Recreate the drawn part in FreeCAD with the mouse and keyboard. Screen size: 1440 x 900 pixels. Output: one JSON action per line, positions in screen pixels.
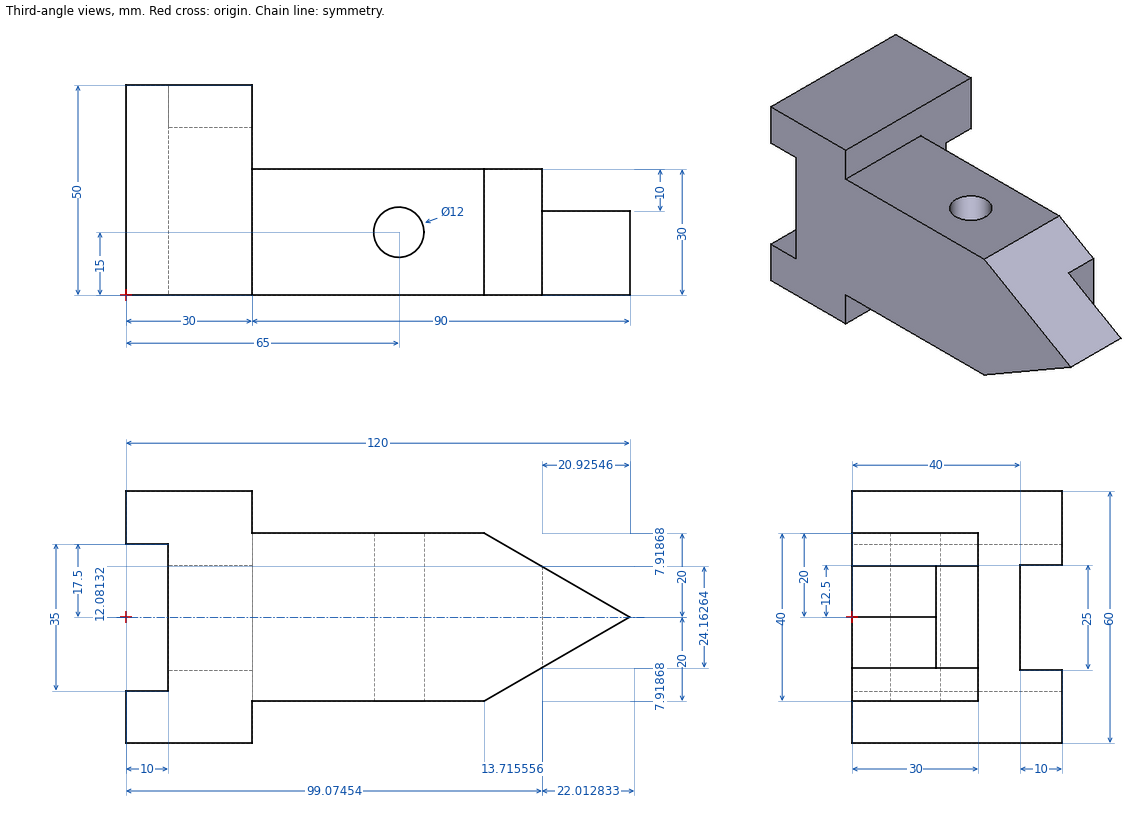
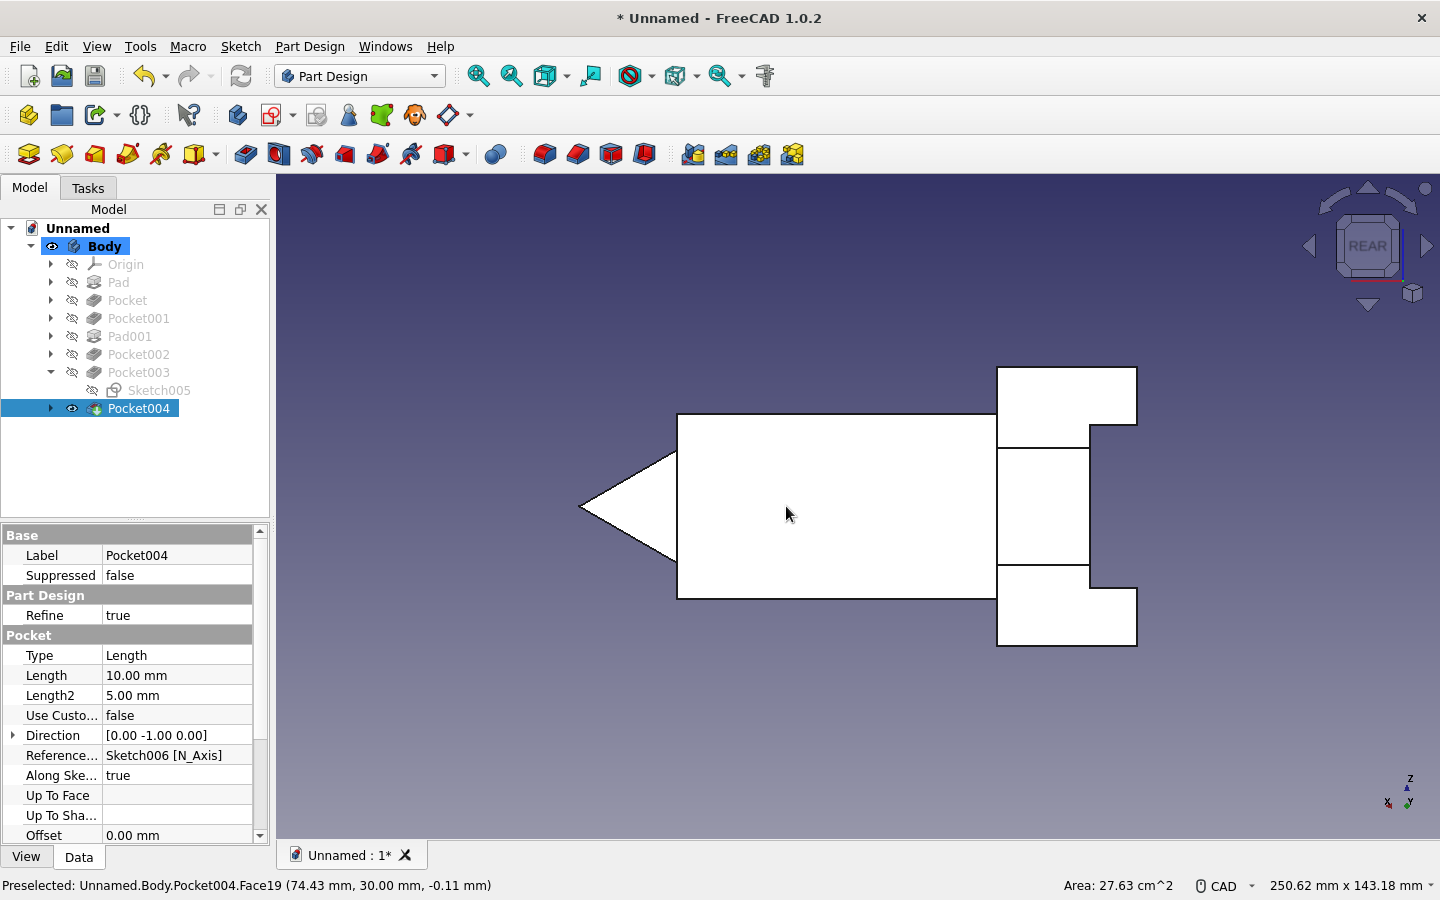
{"action": "left_click", "coordinate": [270, 116]}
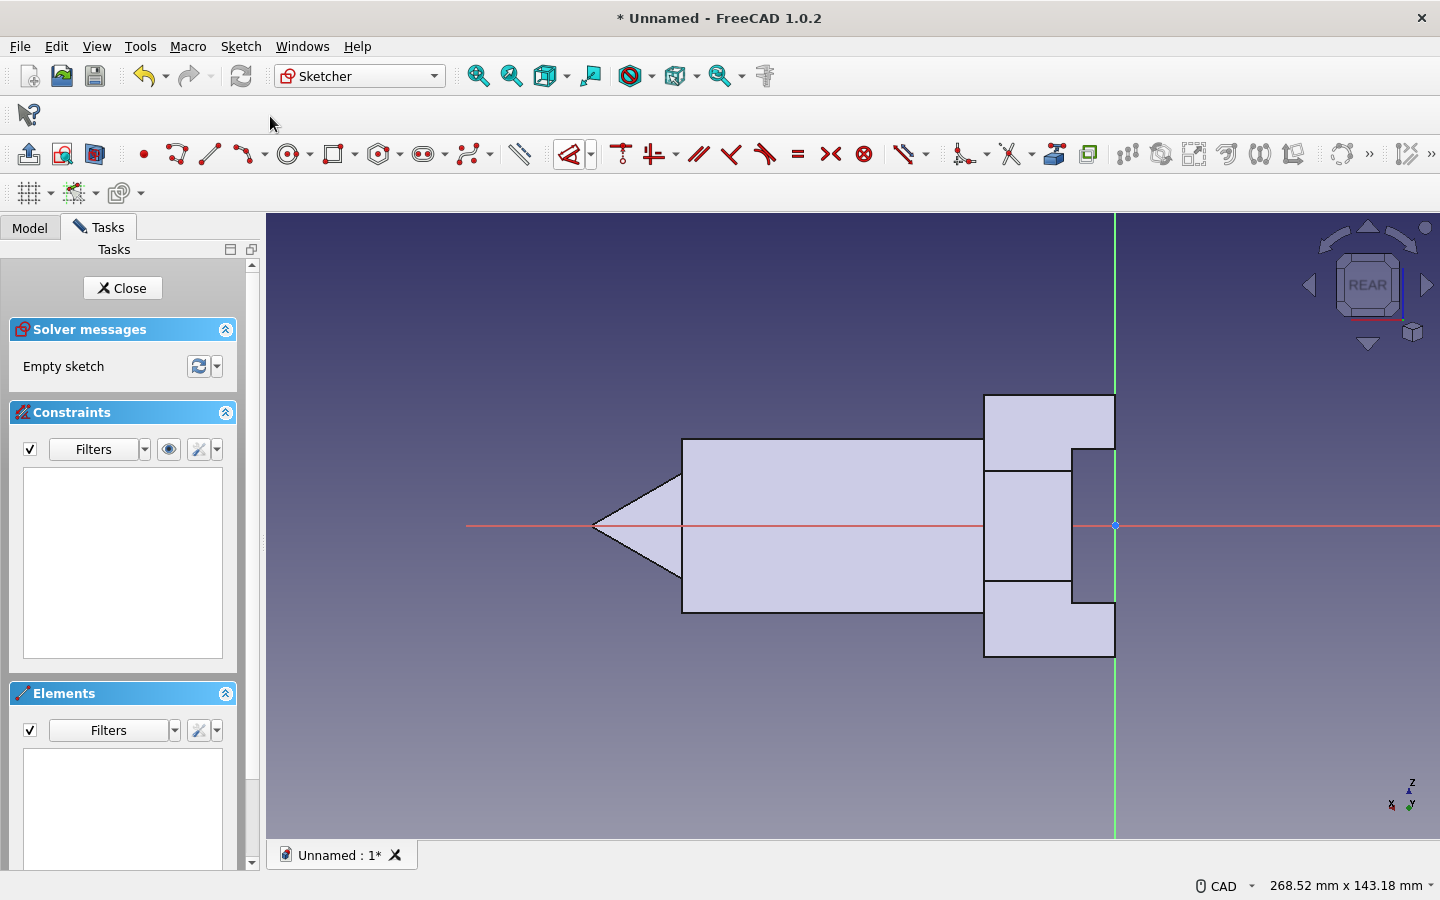
{"action": "scroll", "coordinate": [1131, 526], "scroll_direction": "up", "scroll_amount": 2}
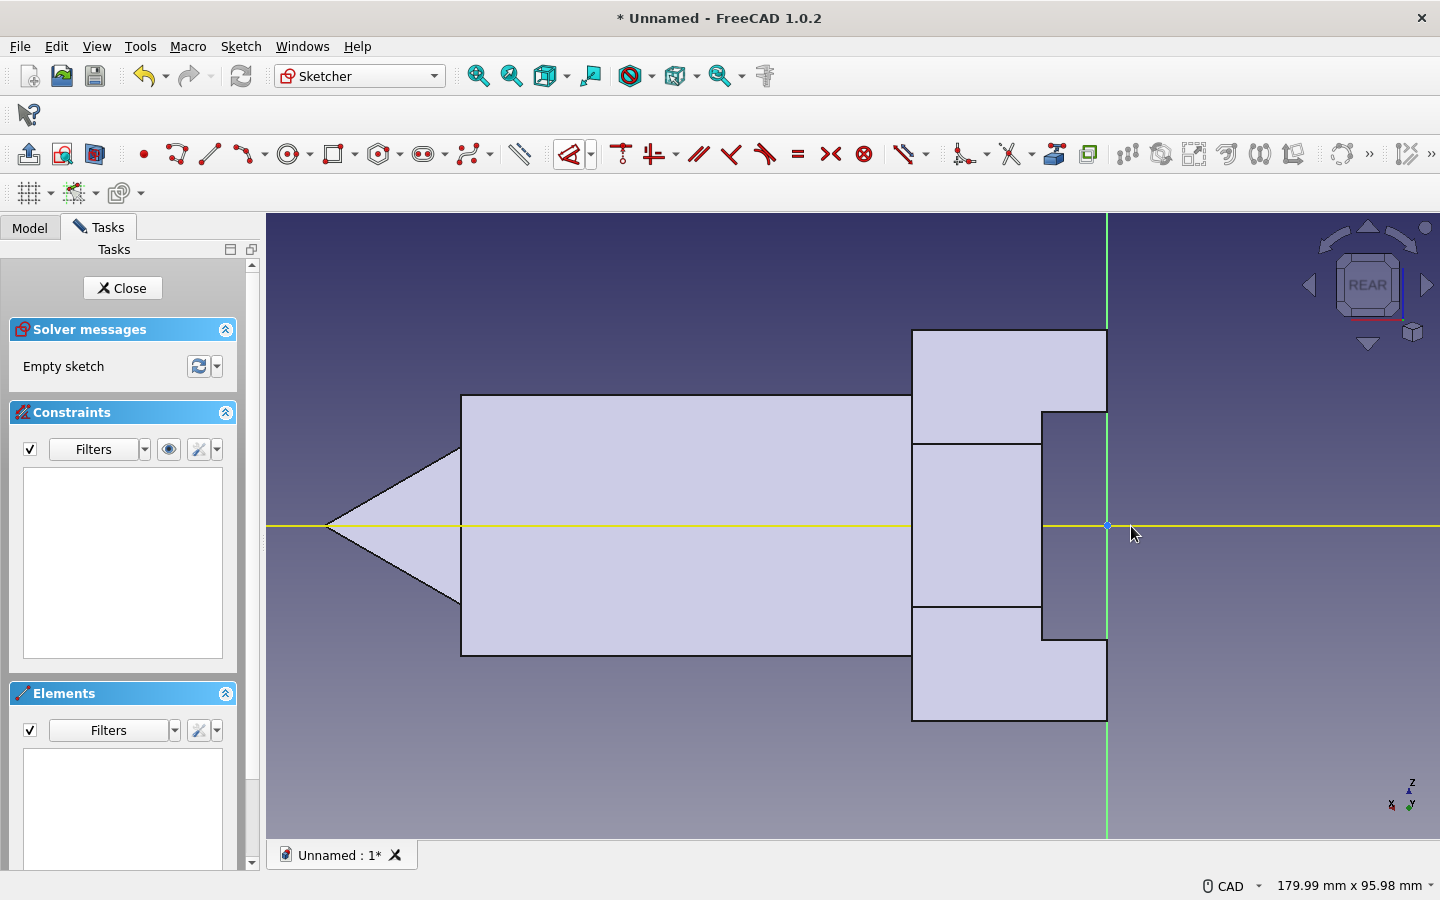
{"action": "key", "text": "g m"}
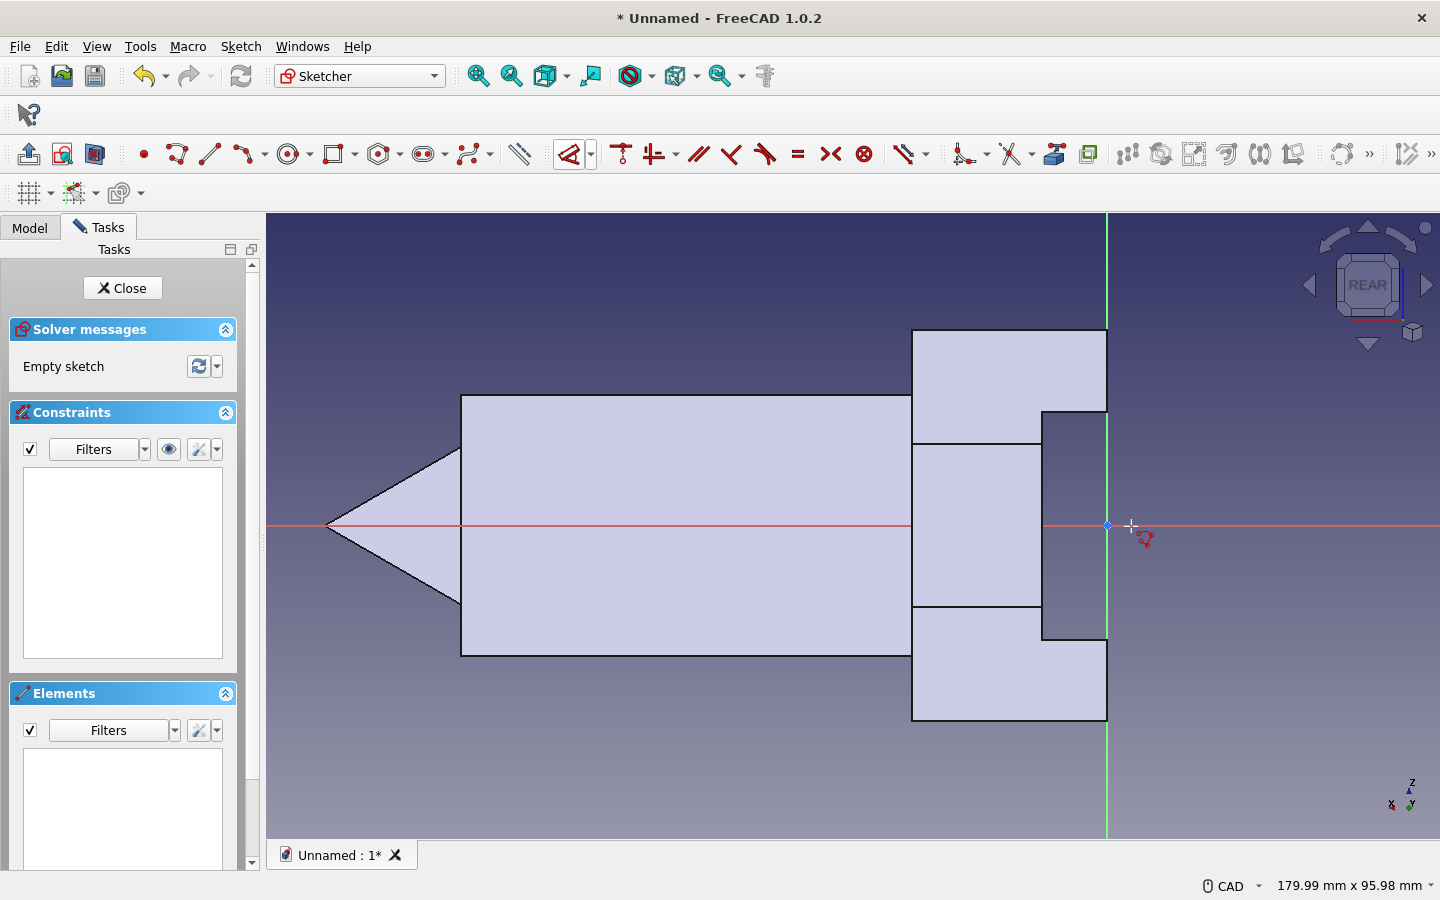
{"action": "left_click", "coordinate": [551, 656]}
{"action": "left_click", "coordinate": [461, 605]}
{"action": "left_click", "coordinate": [461, 656]}
{"action": "left_click", "coordinate": [551, 657]}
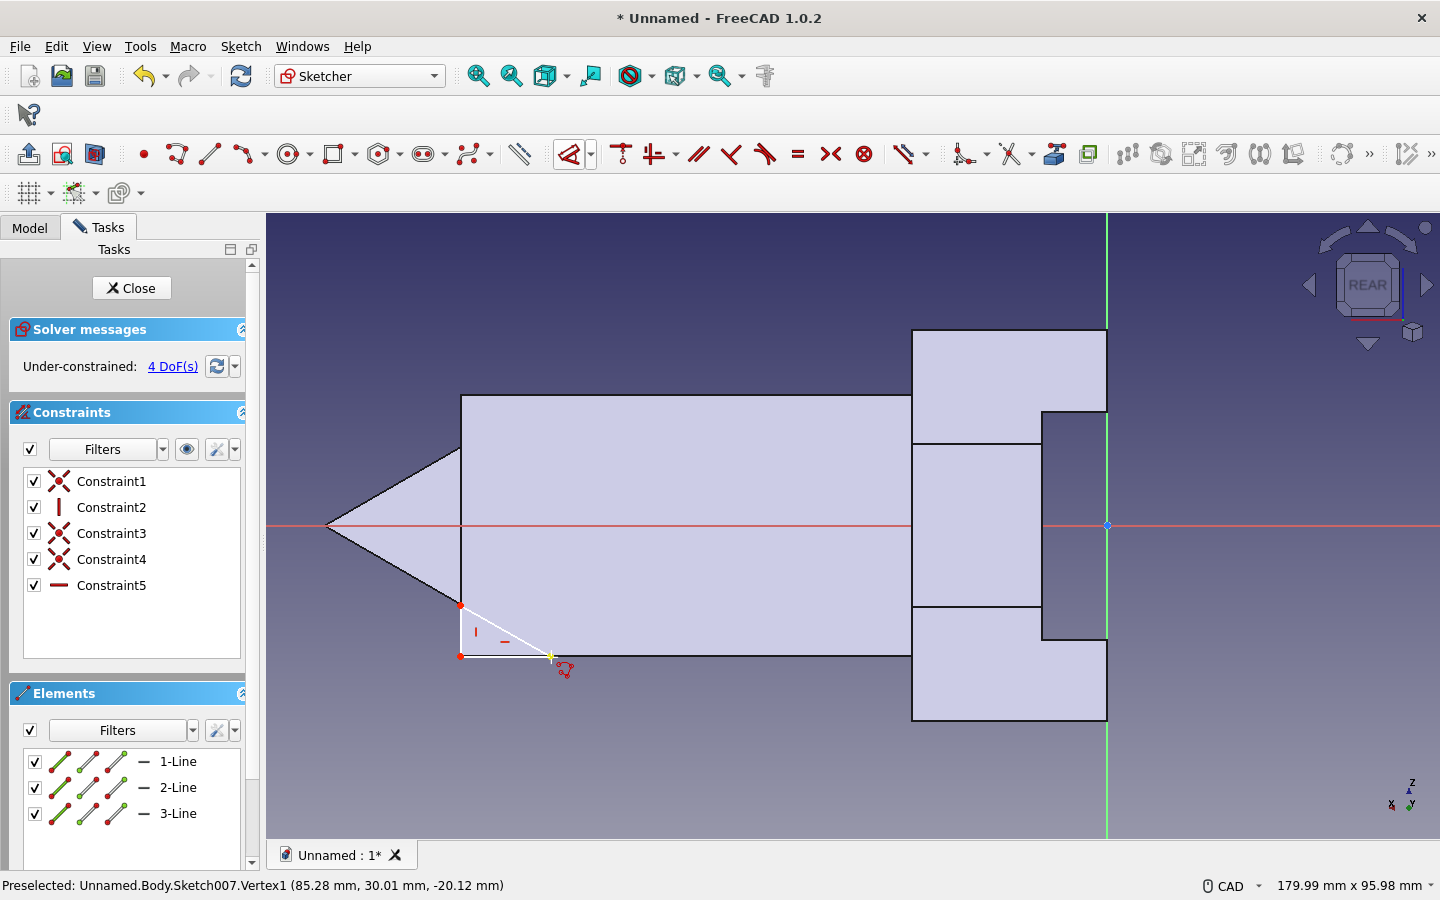
{"action": "left_click", "coordinate": [551, 395]}
{"action": "left_click", "coordinate": [461, 395]}
{"action": "left_click", "coordinate": [461, 447]}
{"action": "left_click", "coordinate": [551, 396]}
{"action": "key", "text": "Escape"}
{"action": "key", "text": "Escape"}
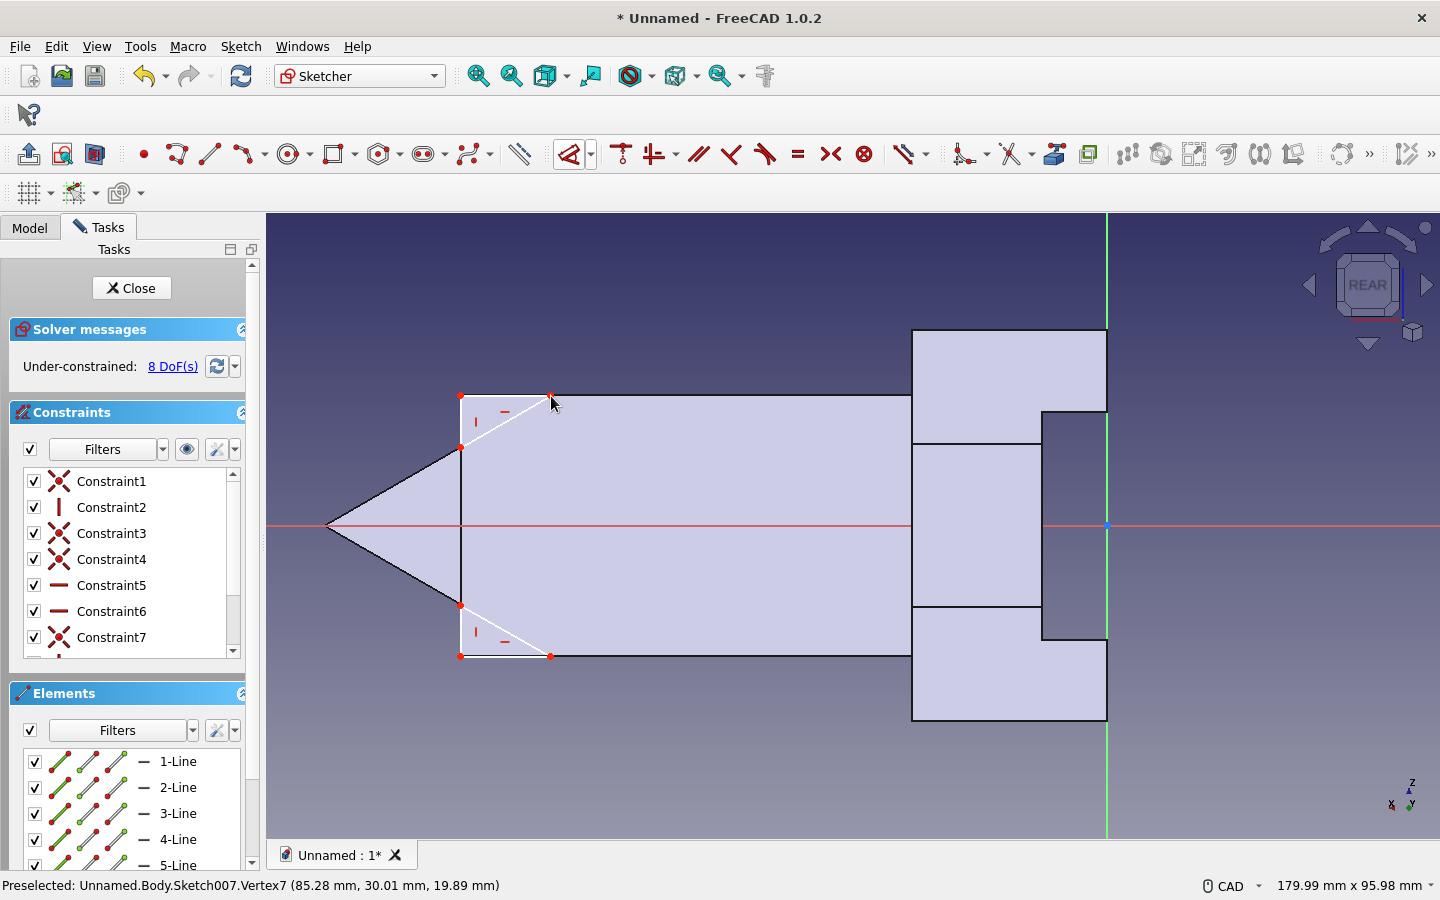
{"action": "left_click", "coordinate": [551, 657]}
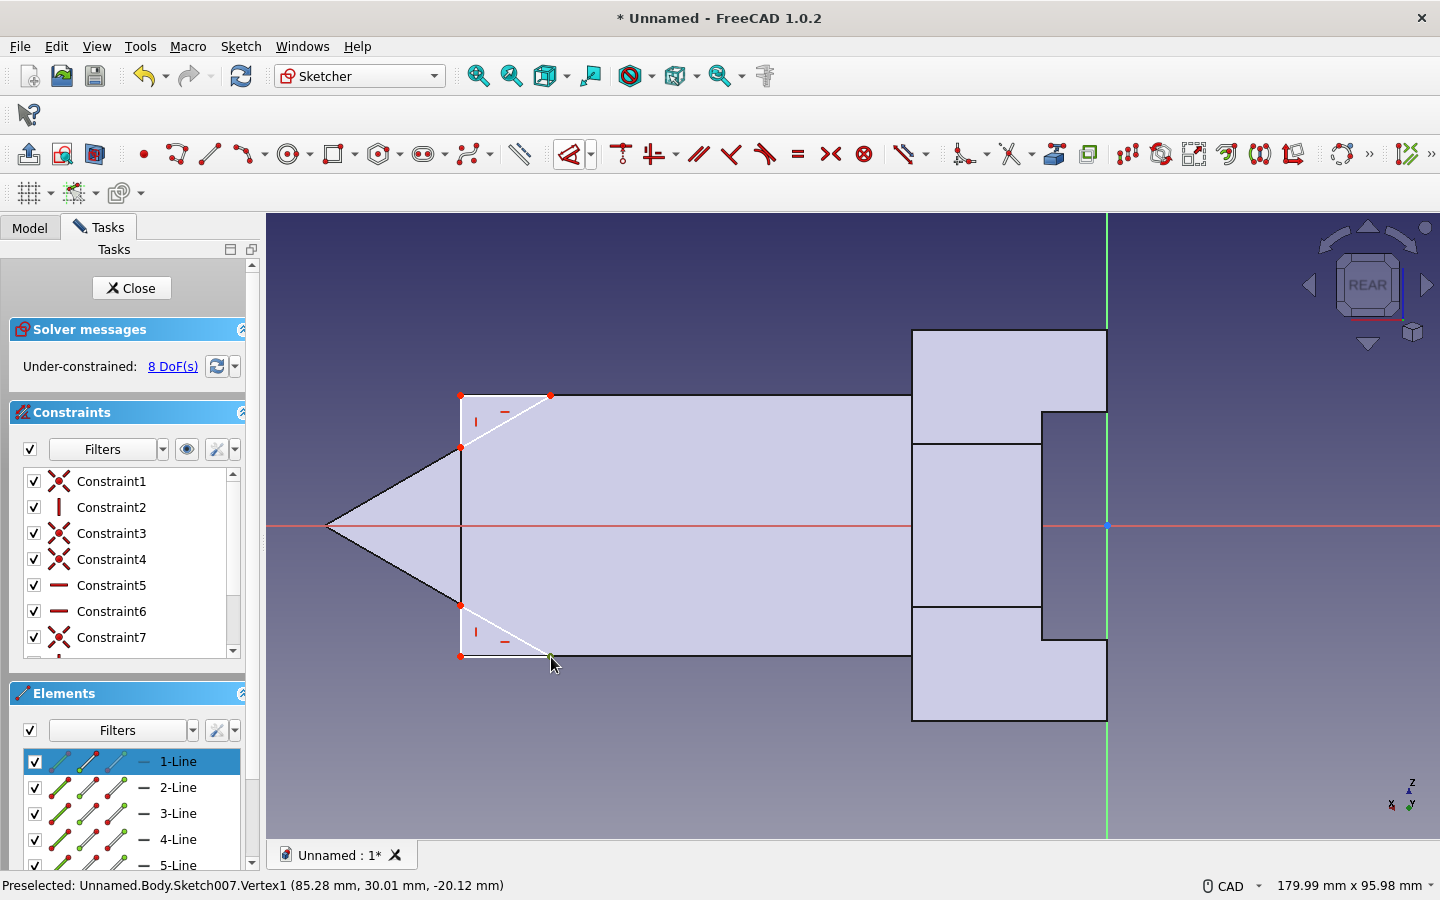
{"action": "left_click", "coordinate": [551, 396]}